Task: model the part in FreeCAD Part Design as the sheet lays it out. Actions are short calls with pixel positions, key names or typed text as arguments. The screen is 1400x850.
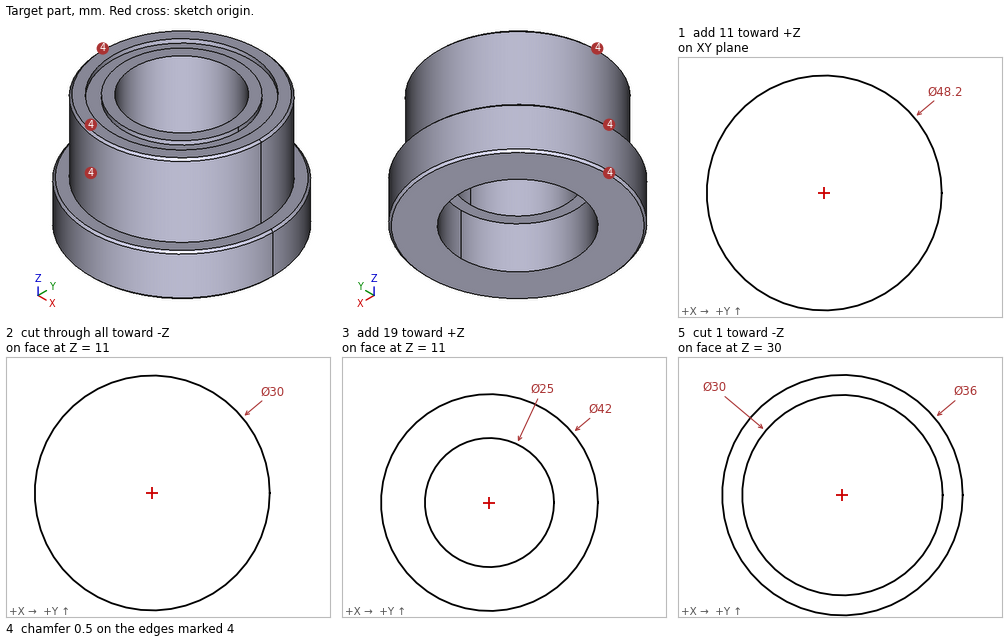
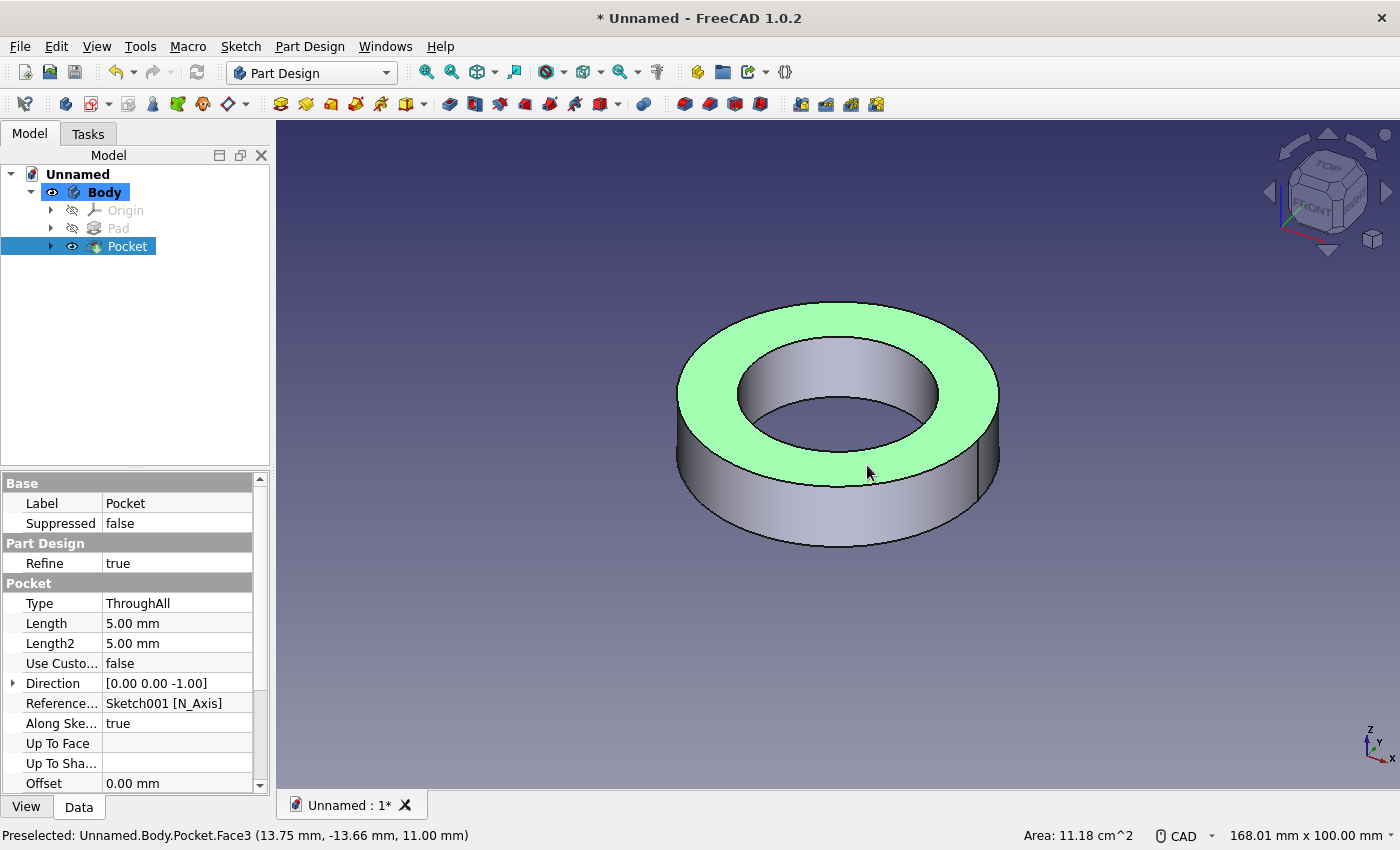
click(90, 104)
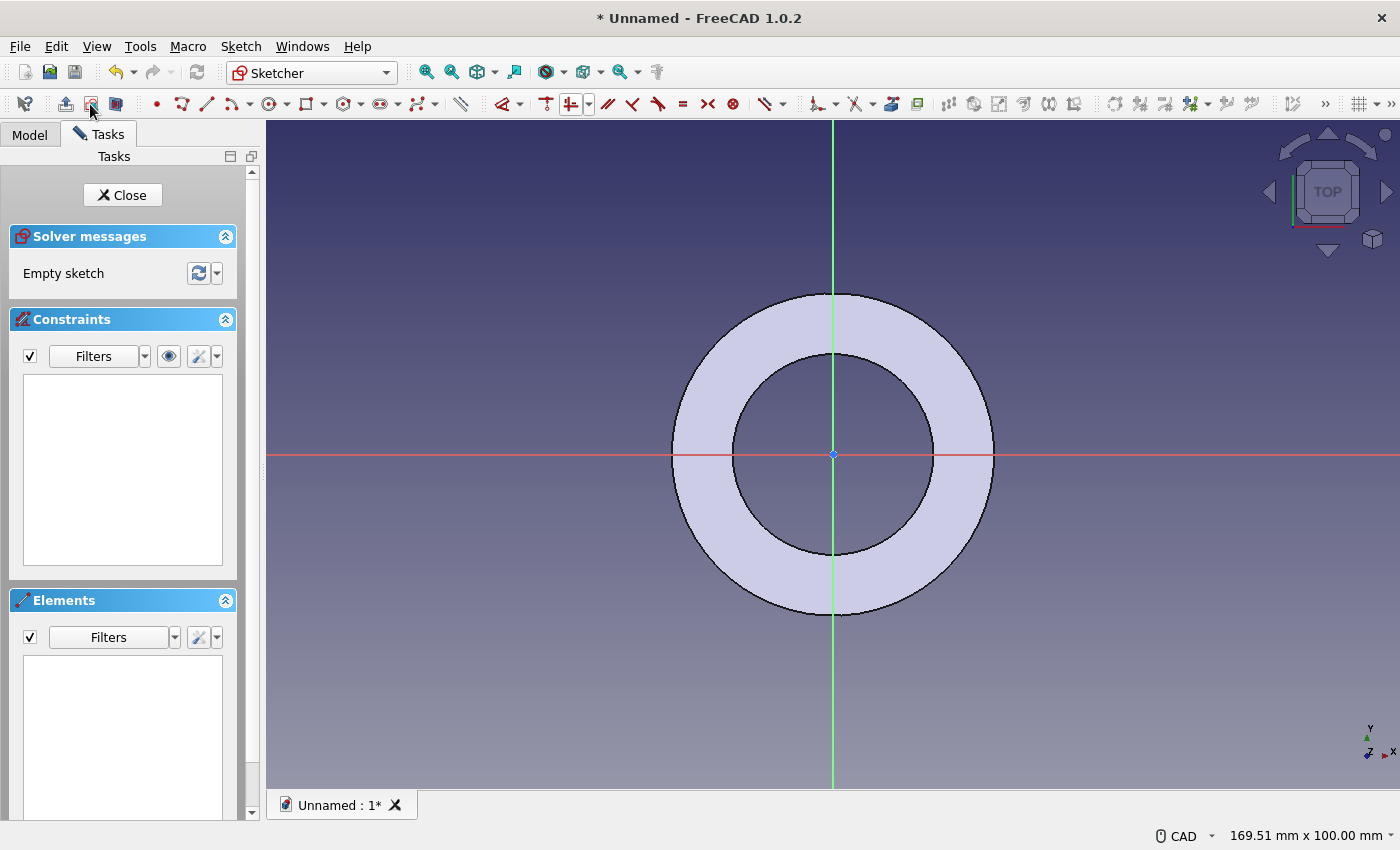
scroll(972, 455, up, 2)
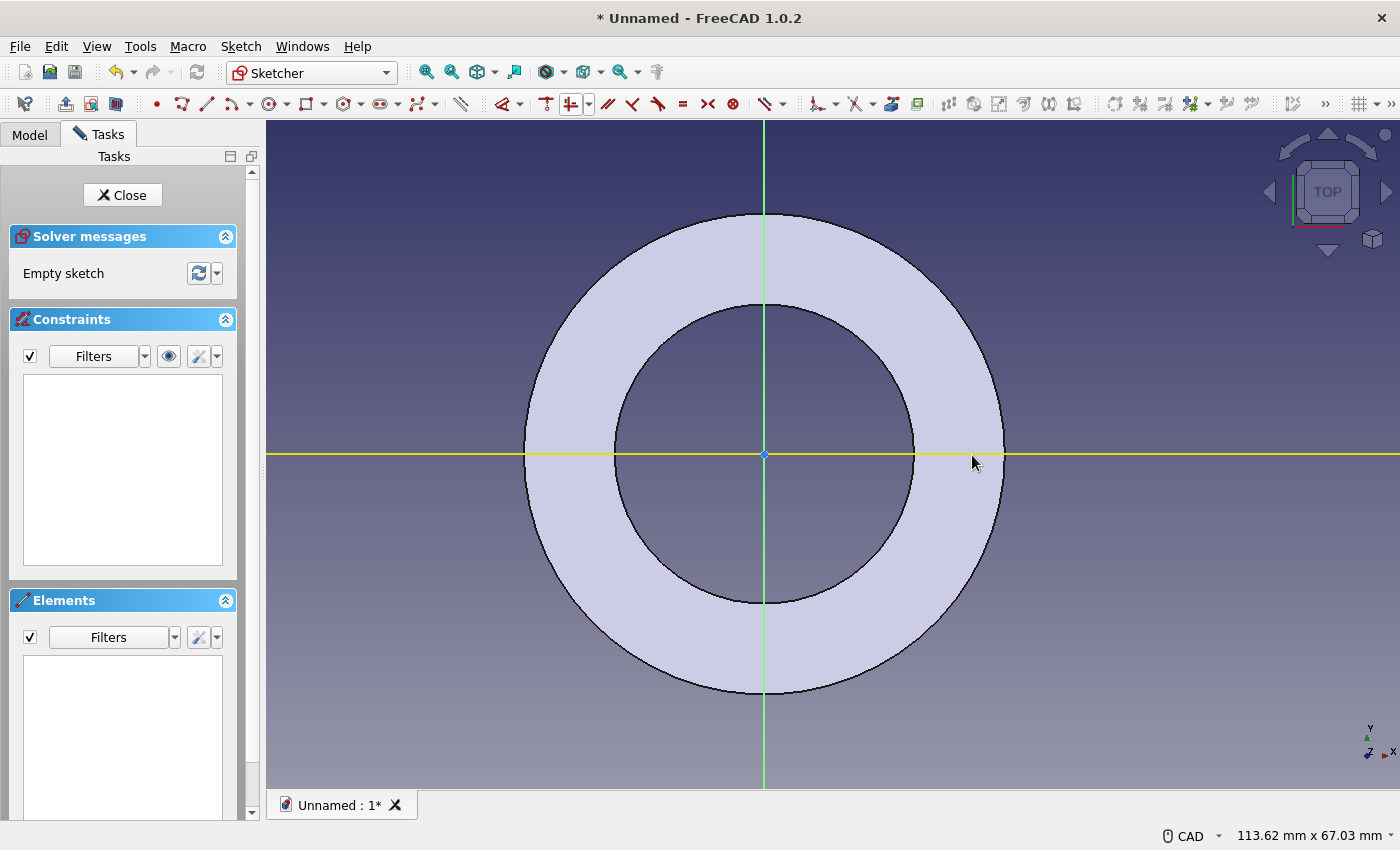
key(g)
key(c)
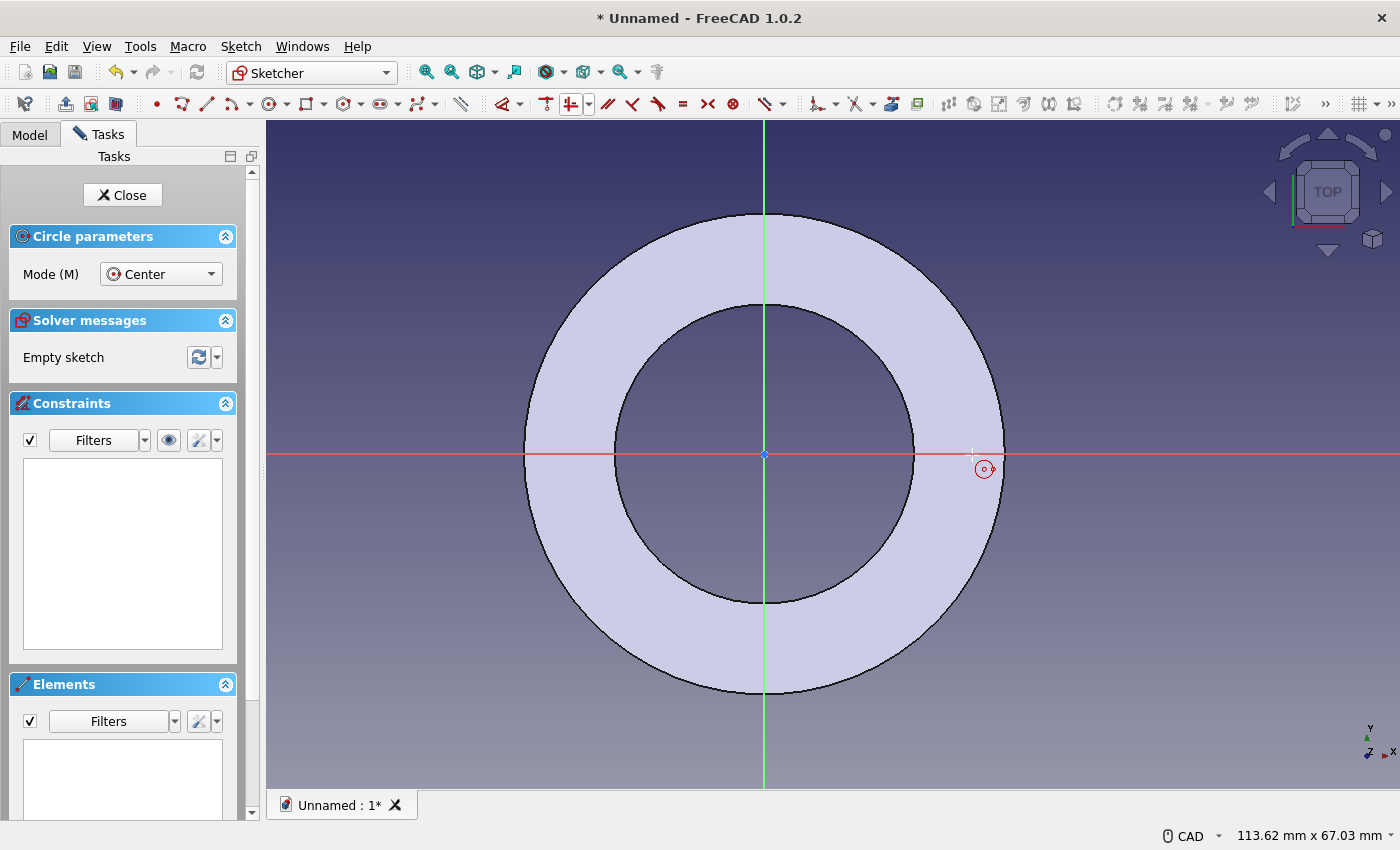
click(764, 454)
click(913, 306)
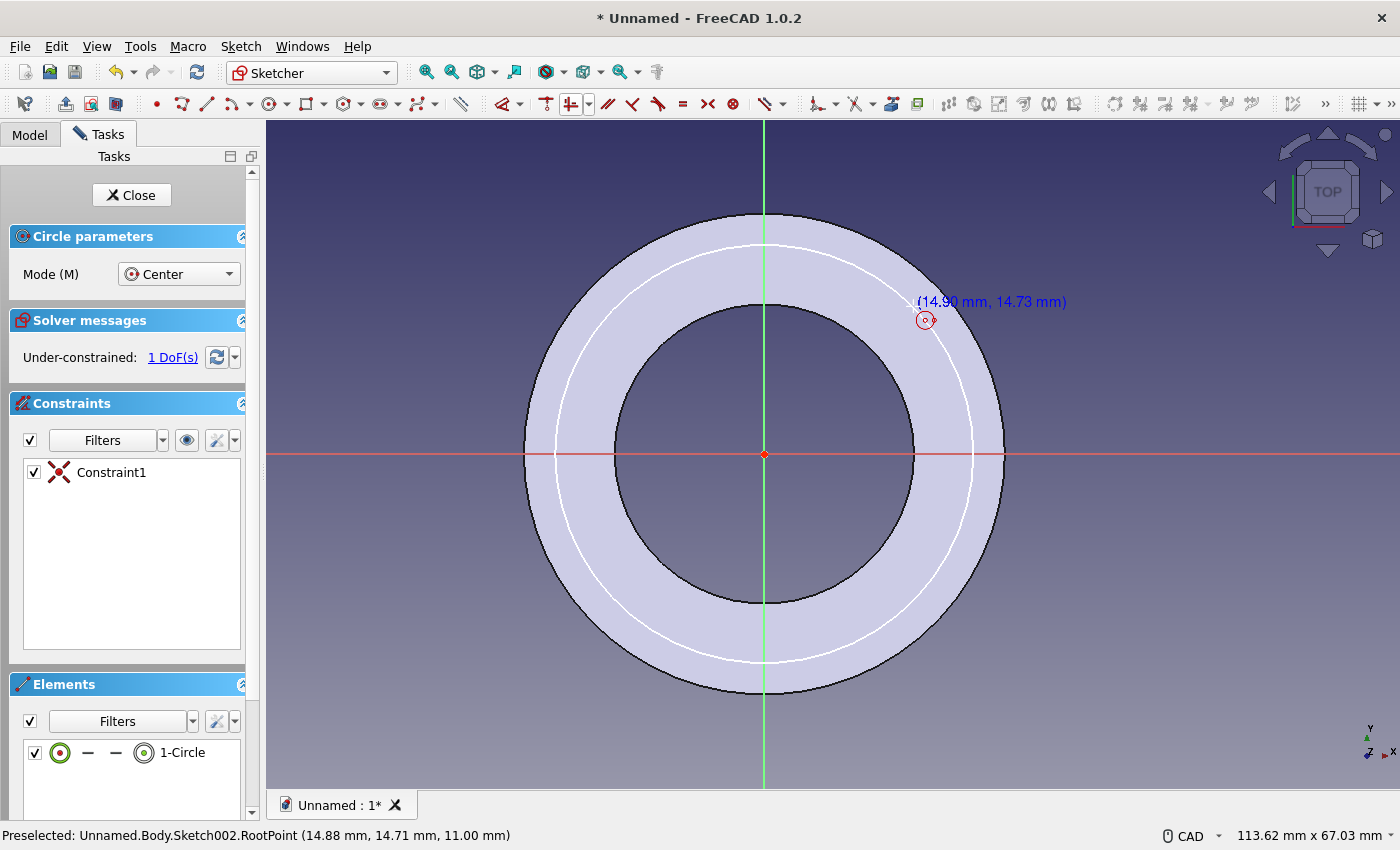
click(764, 454)
click(853, 366)
key(Escape)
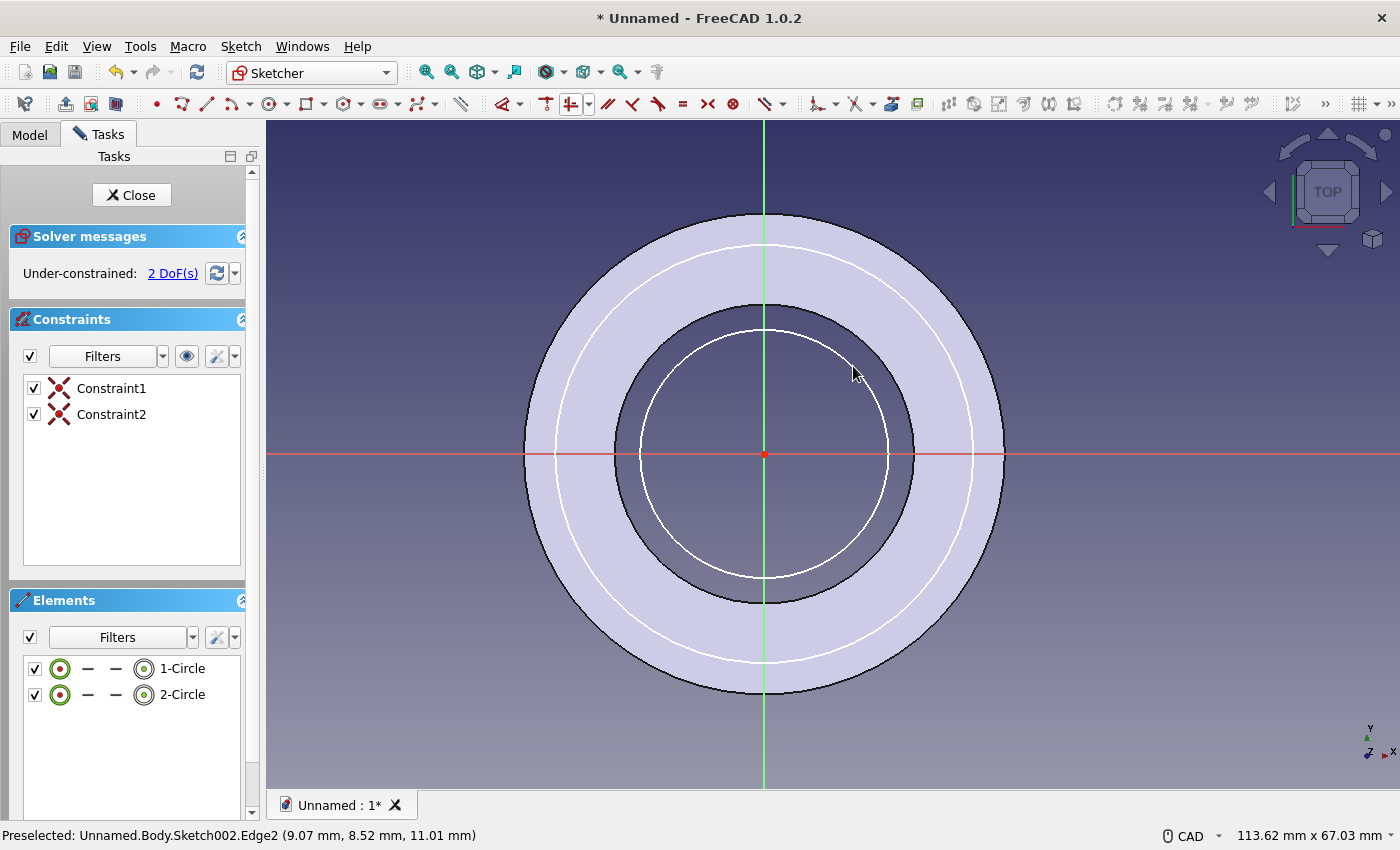
key(d)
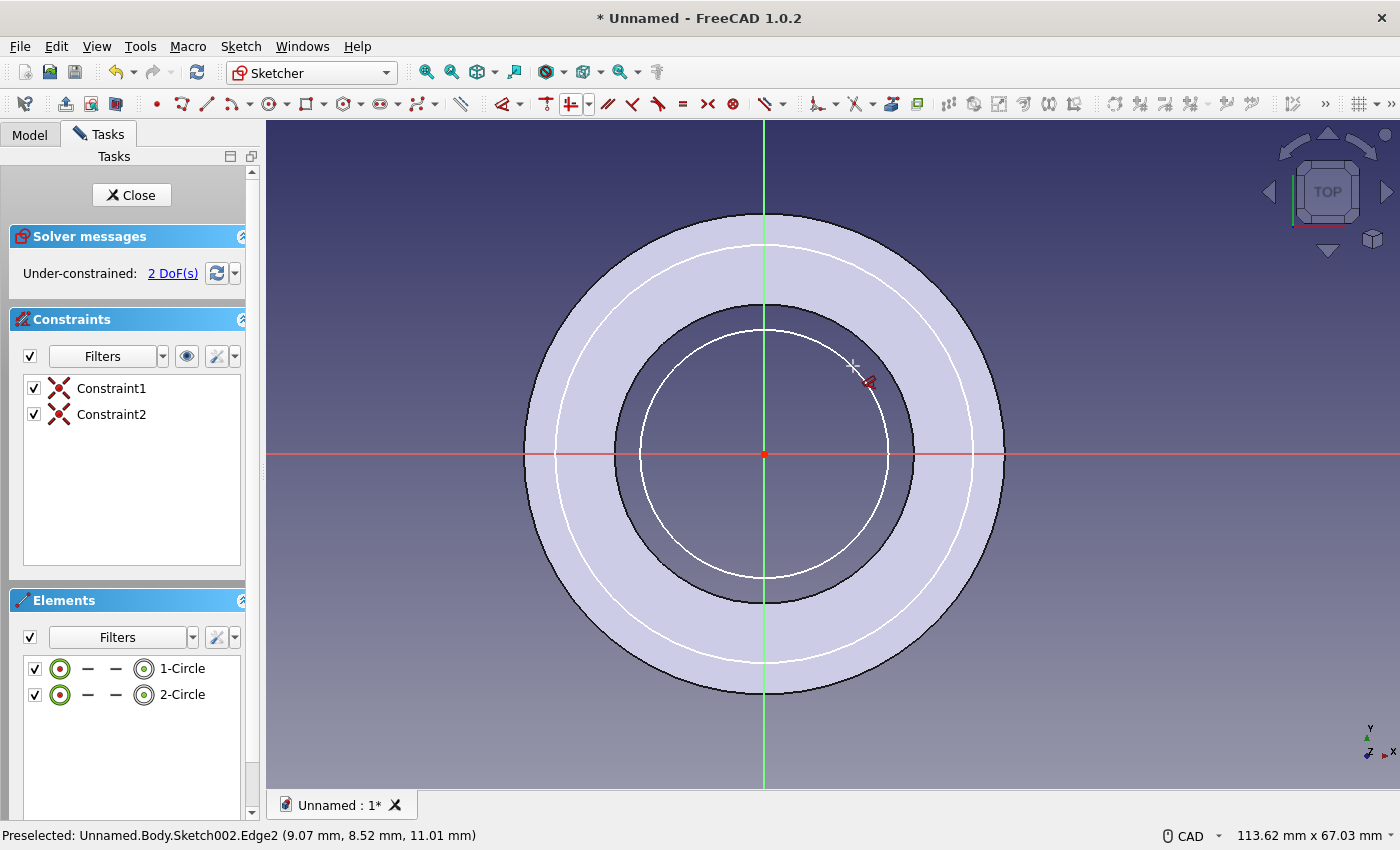
click(912, 306)
click(935, 283)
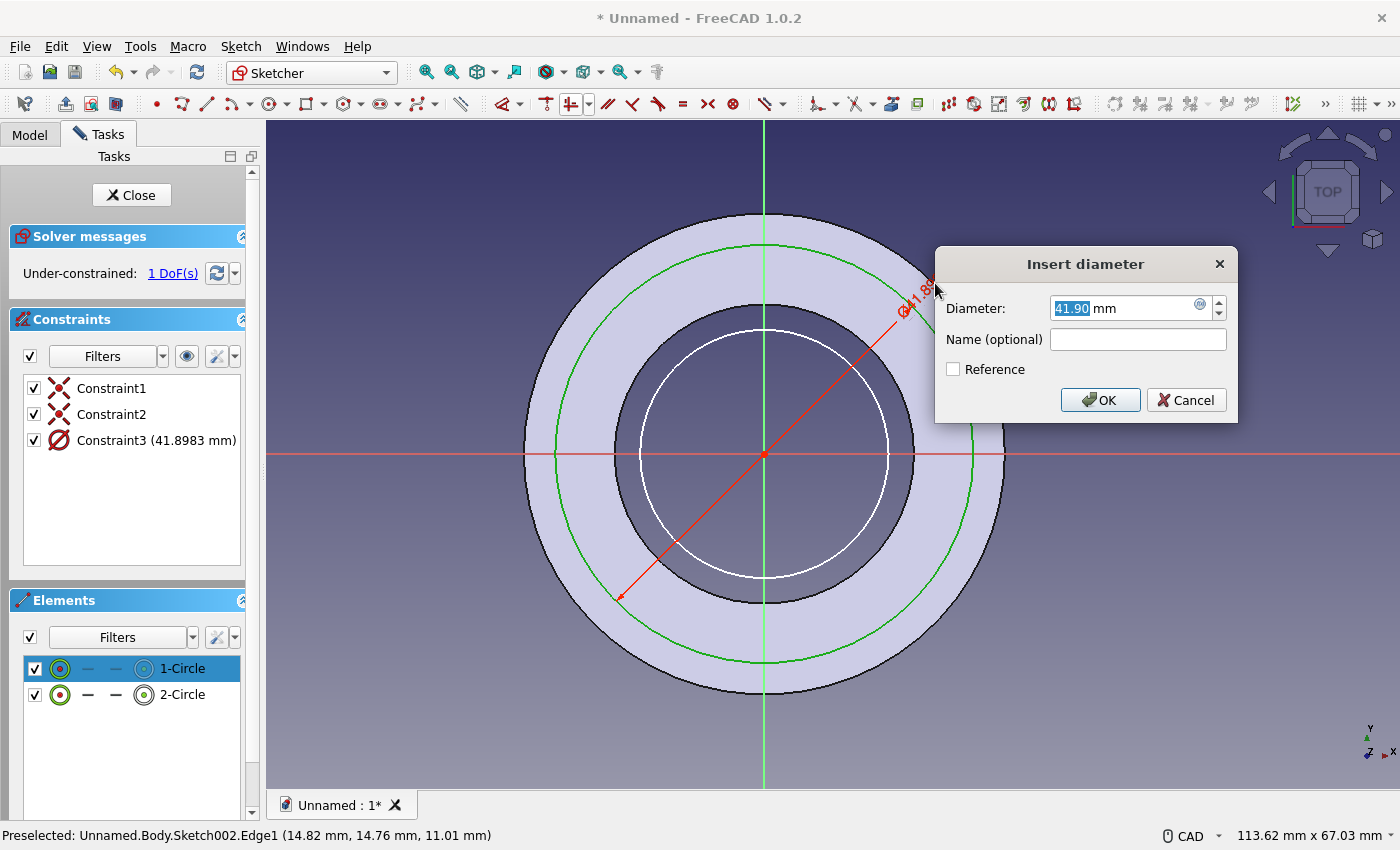
text(42)
key(Return)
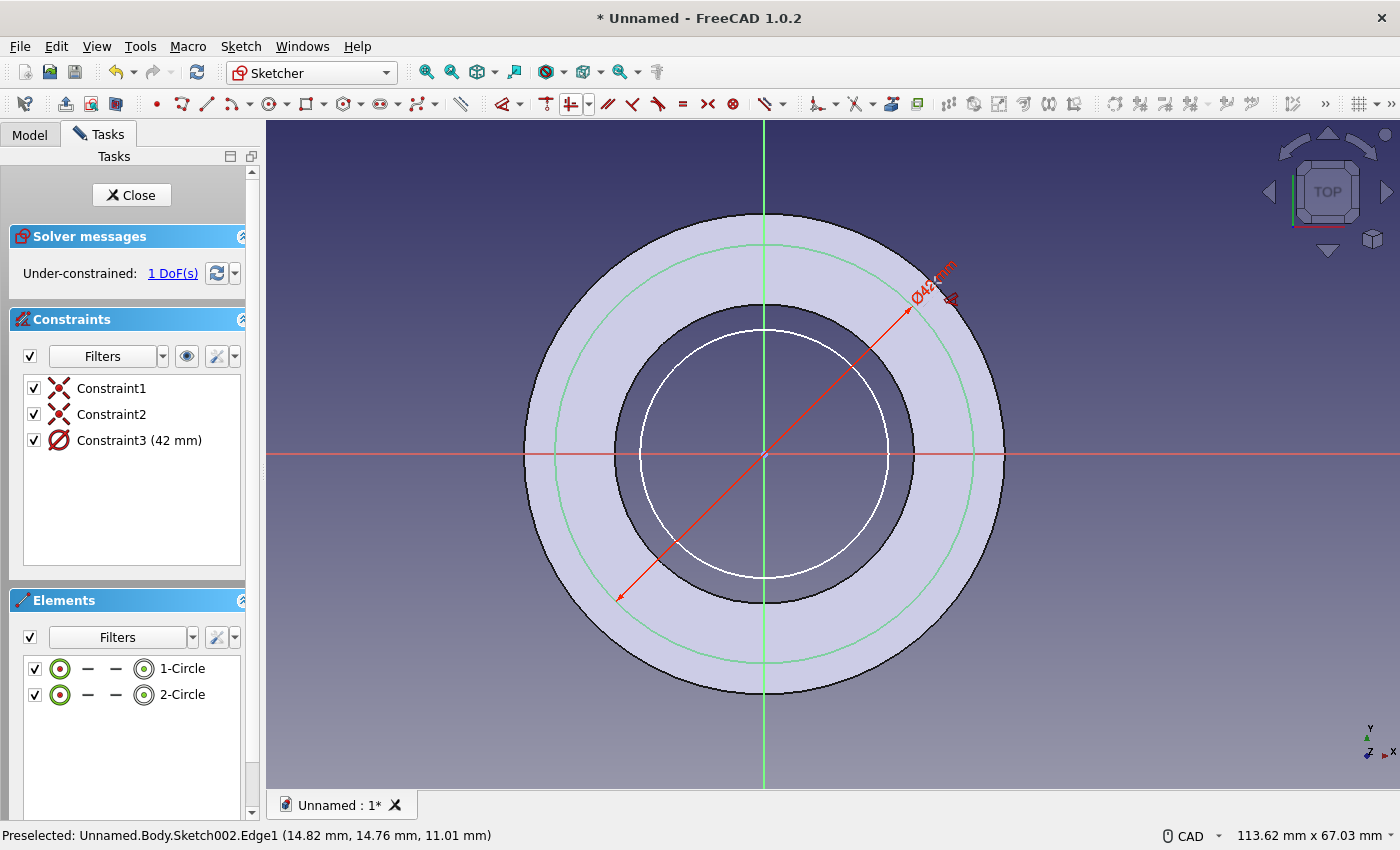
click(852, 366)
click(875, 343)